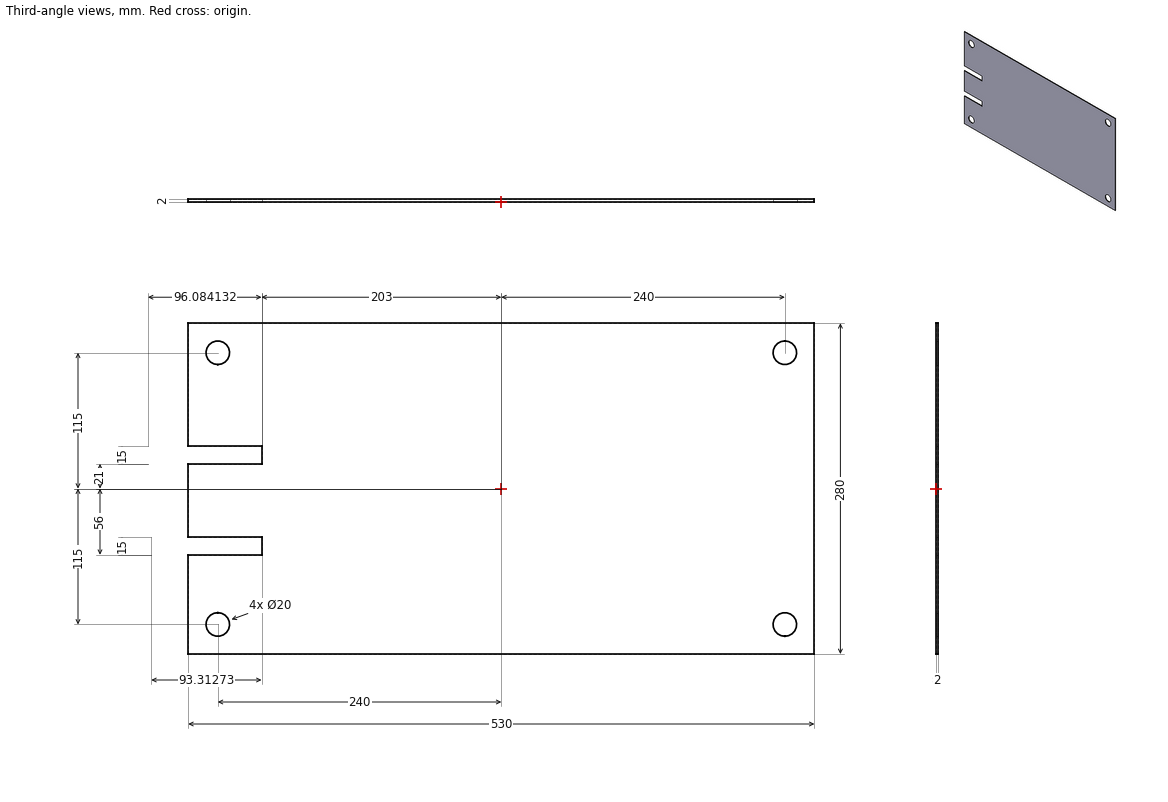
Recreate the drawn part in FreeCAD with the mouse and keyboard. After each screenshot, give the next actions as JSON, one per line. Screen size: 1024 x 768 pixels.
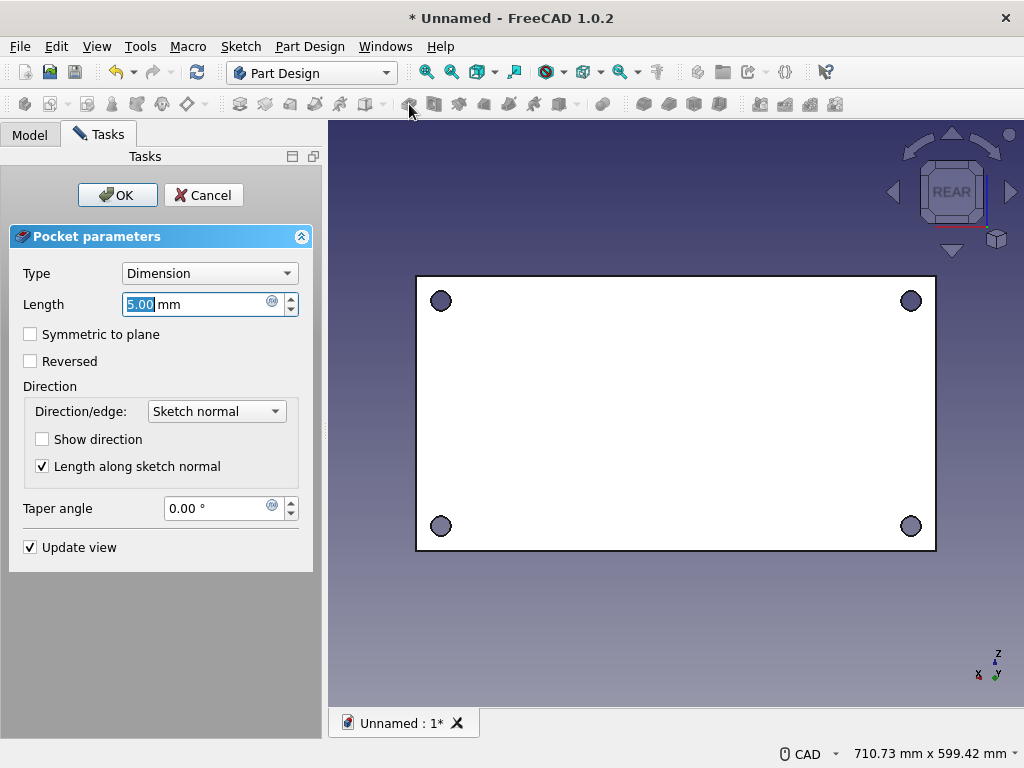
{"action": "type", "text": "2"}
{"action": "key", "text": "Tab"}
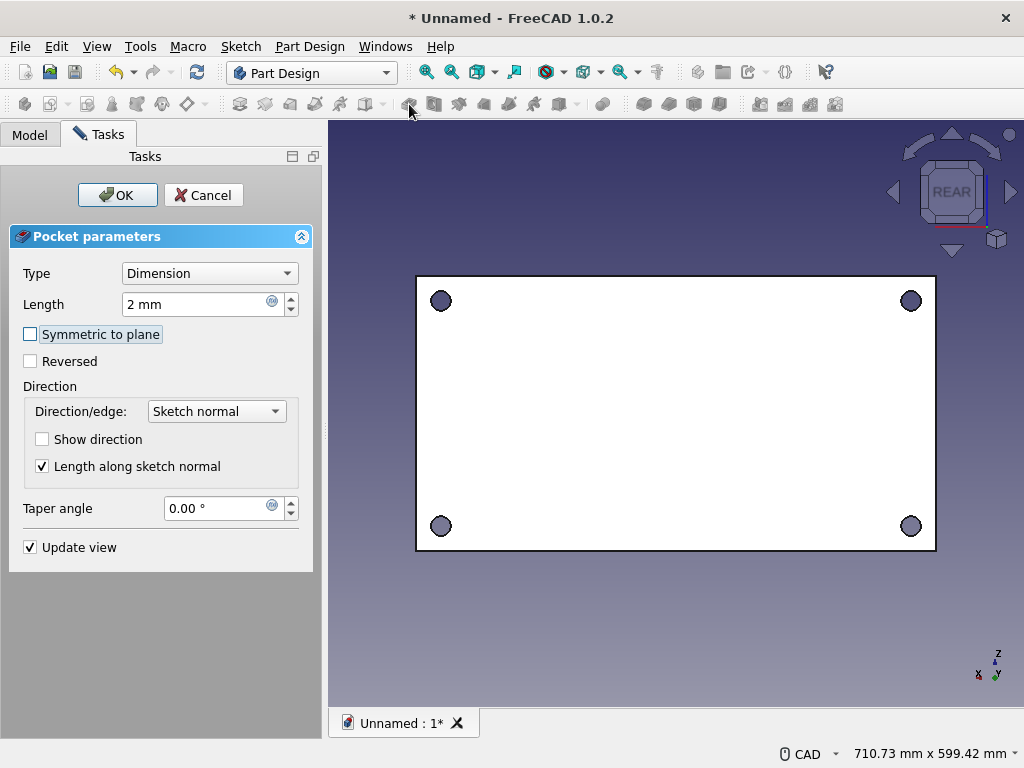
{"action": "left_click", "coordinate": [118, 195]}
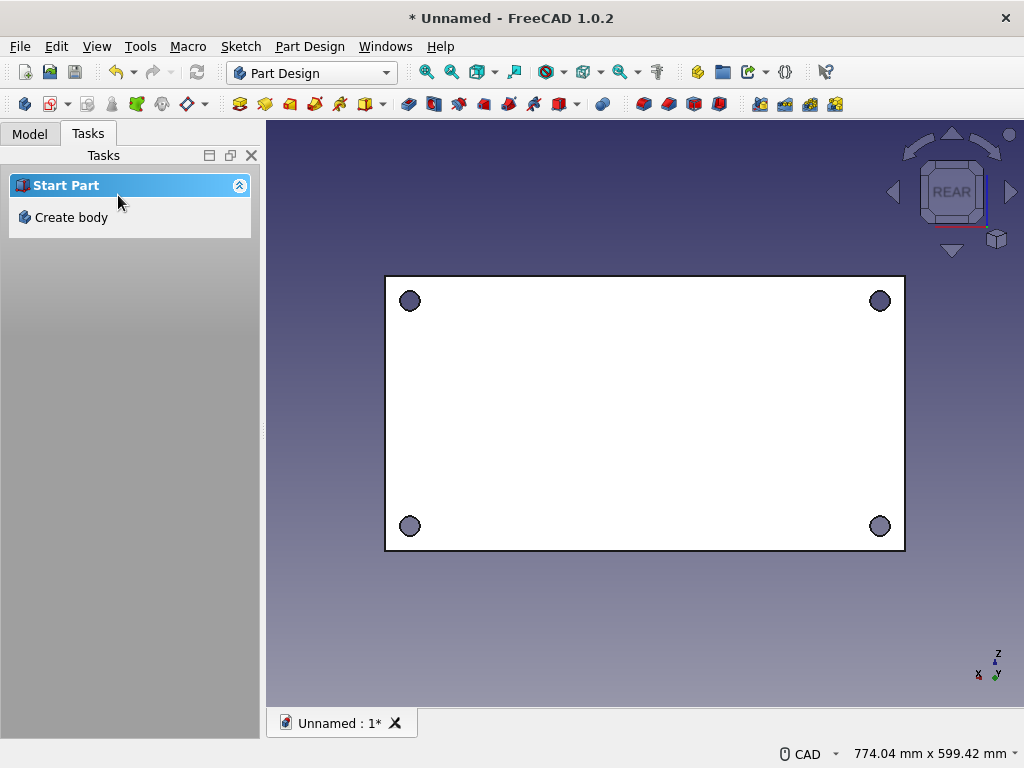
{"action": "left_click", "coordinate": [571, 412]}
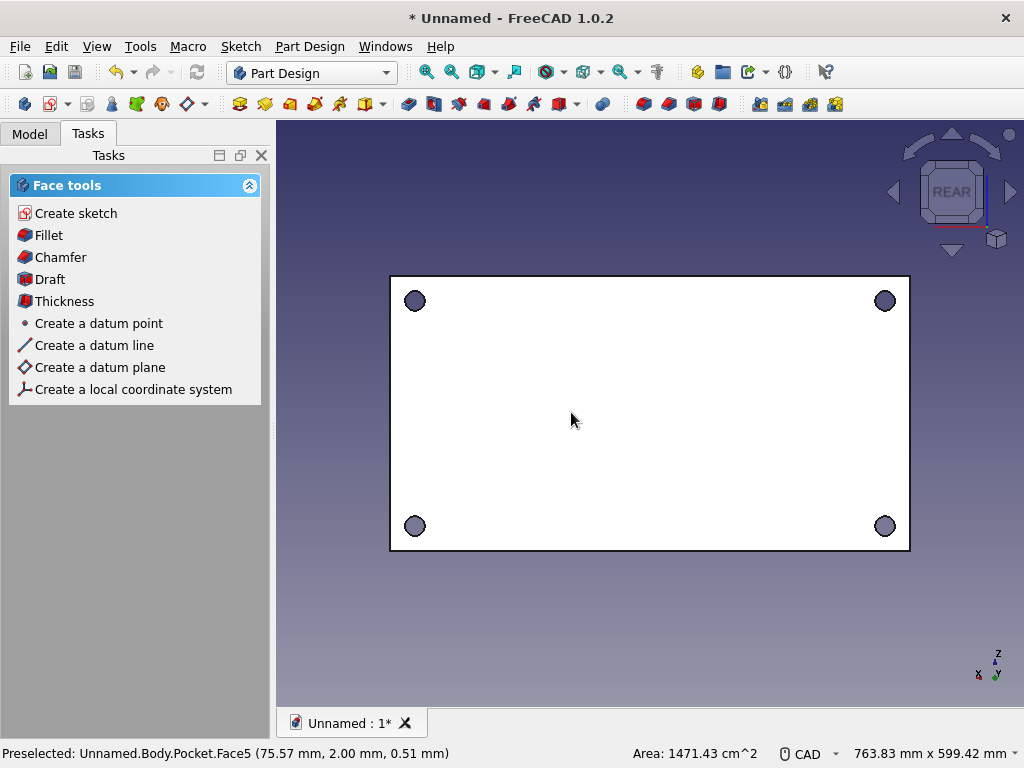
{"action": "left_click", "coordinate": [50, 104]}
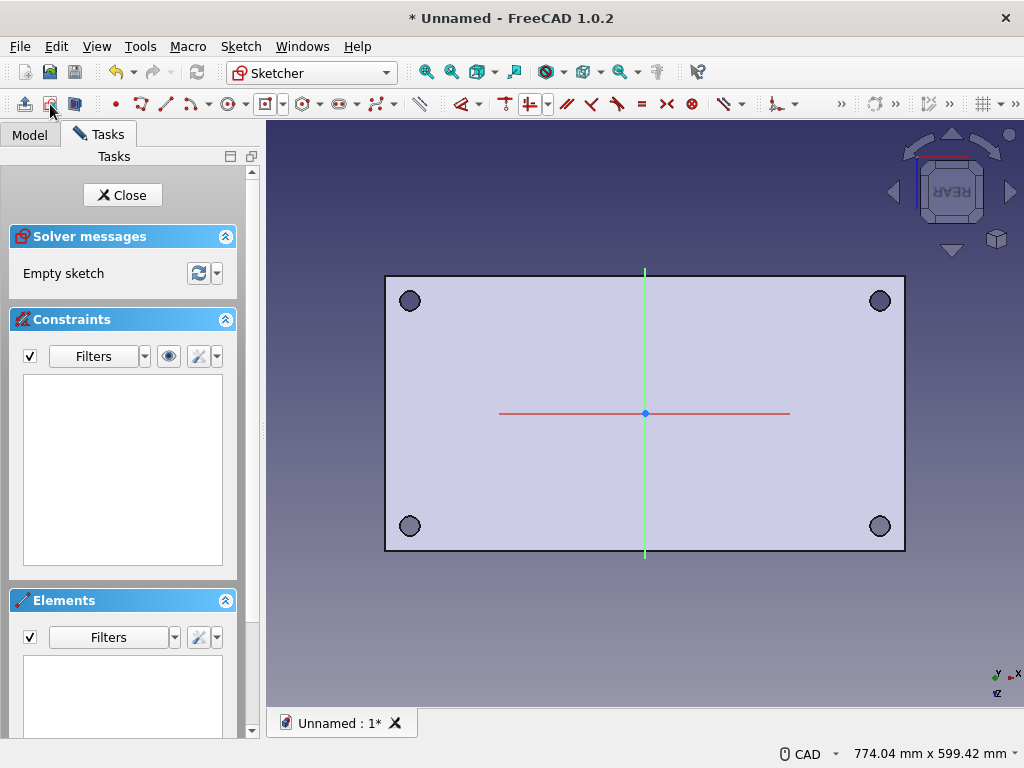
{"action": "scroll", "coordinate": [341, 401], "scroll_direction": "up", "scroll_amount": 7}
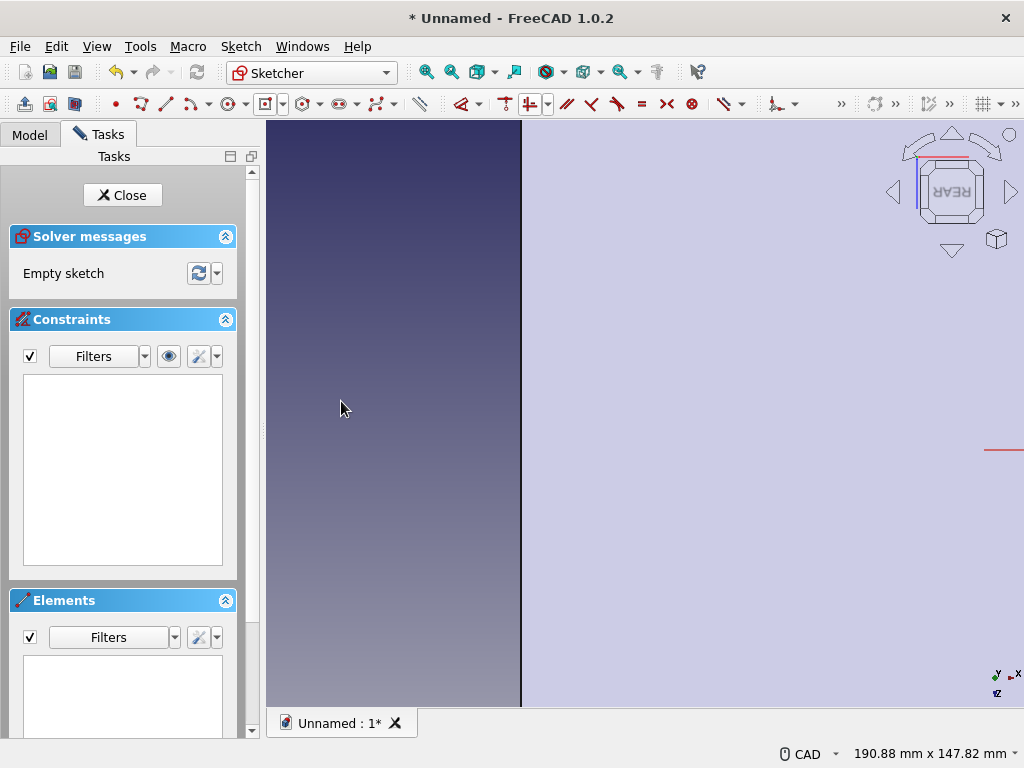
{"action": "key", "text": "g r"}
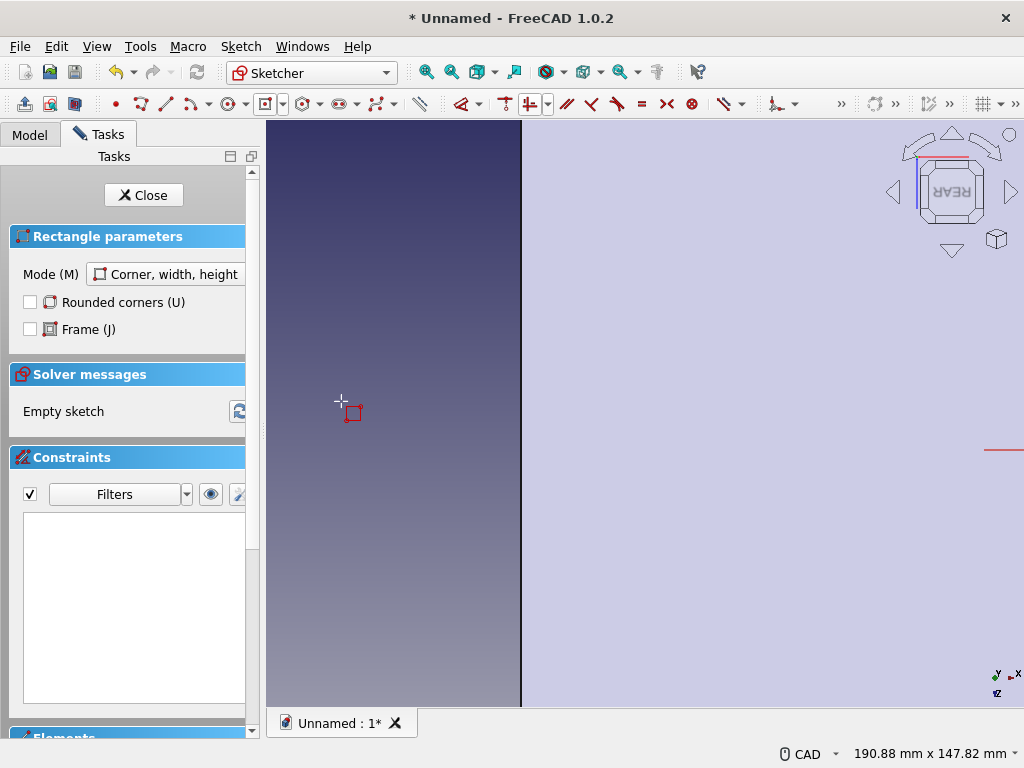
{"action": "left_click", "coordinate": [386, 534]}
{"action": "left_click", "coordinate": [767, 593]}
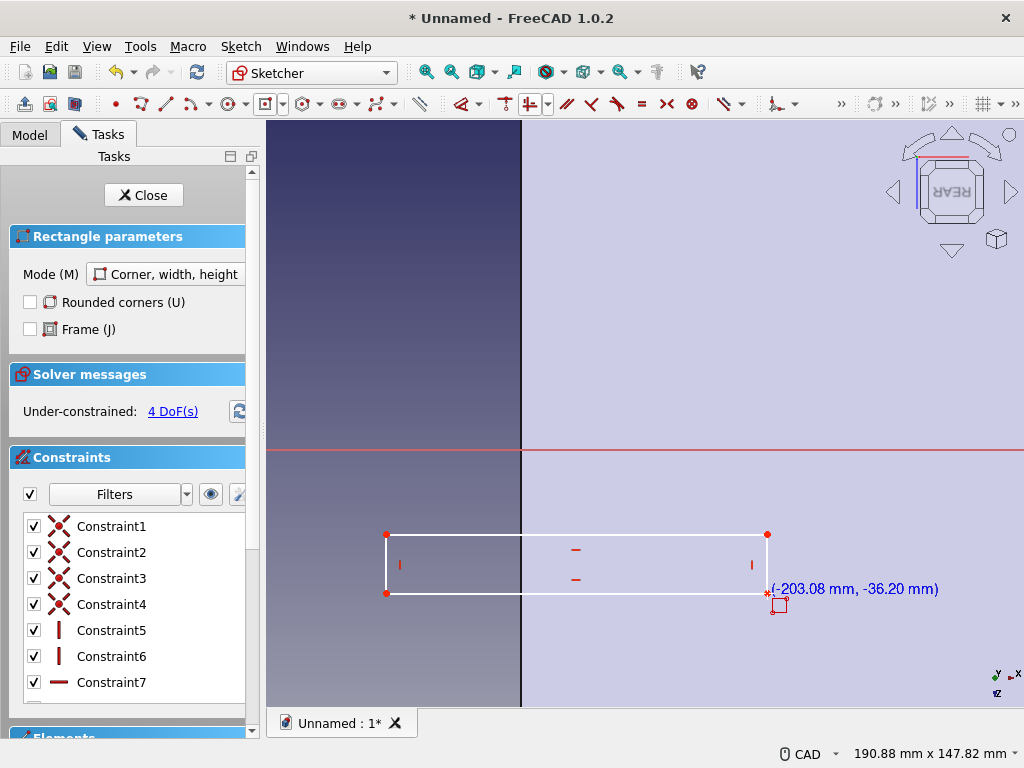
{"action": "left_click", "coordinate": [397, 228]}
{"action": "left_click", "coordinate": [767, 287]}
{"action": "key", "text": "Escape"}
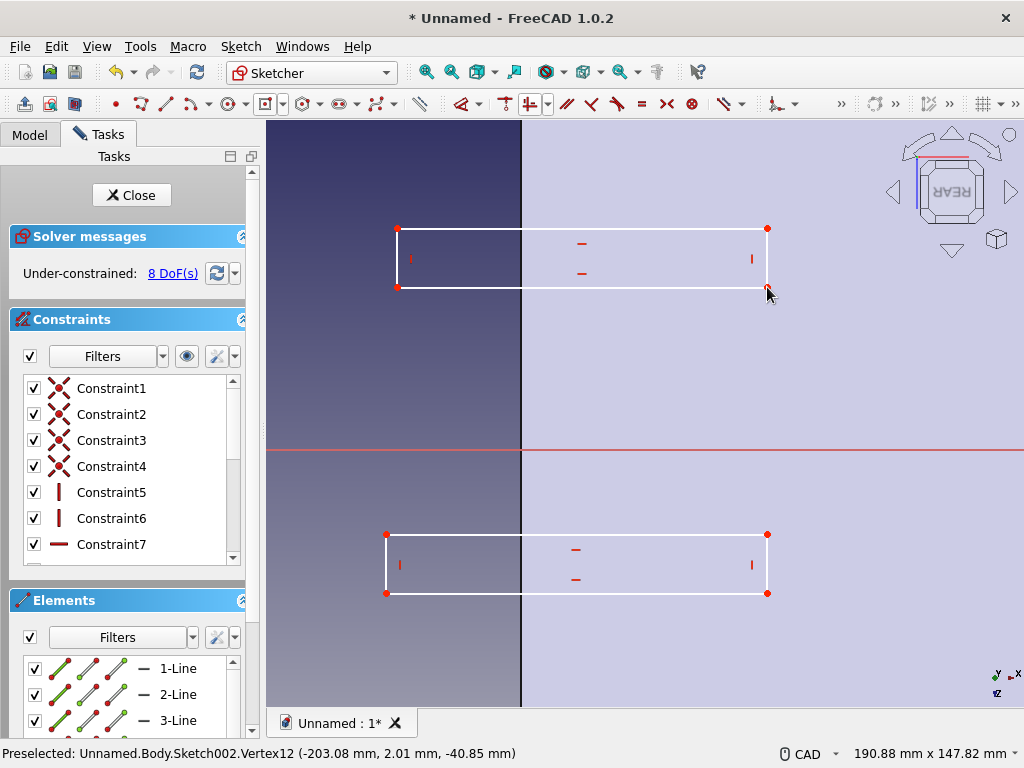
{"action": "left_click", "coordinate": [460, 104]}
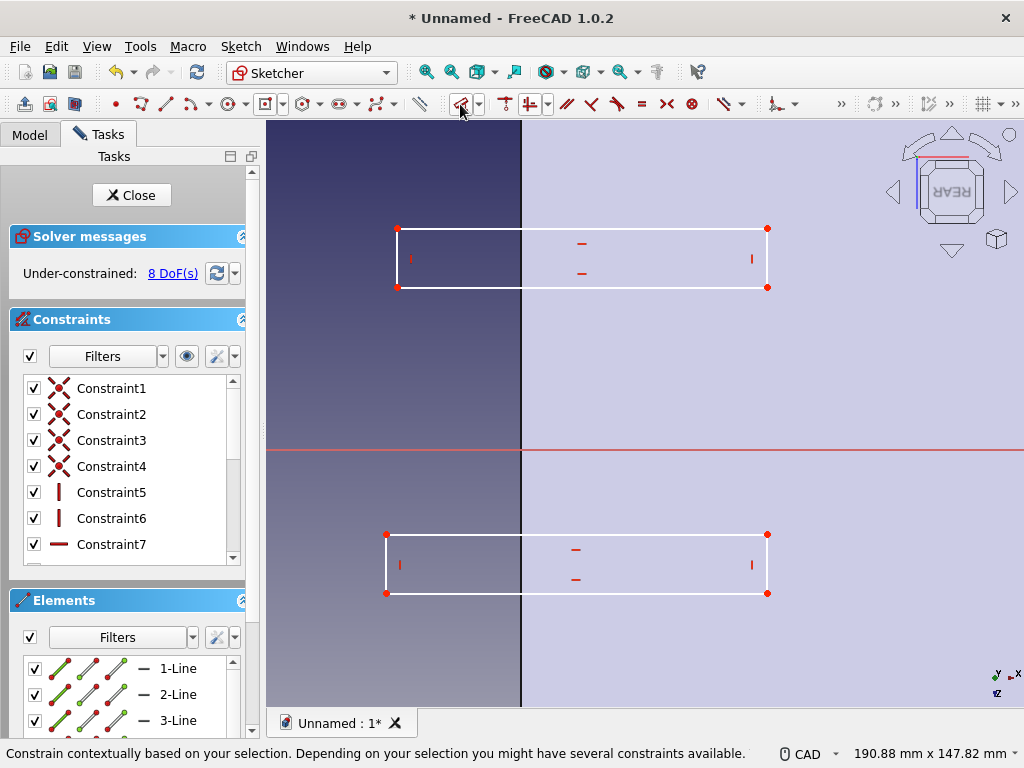
{"action": "left_click", "coordinate": [386, 553]}
{"action": "left_click", "coordinate": [352, 565]}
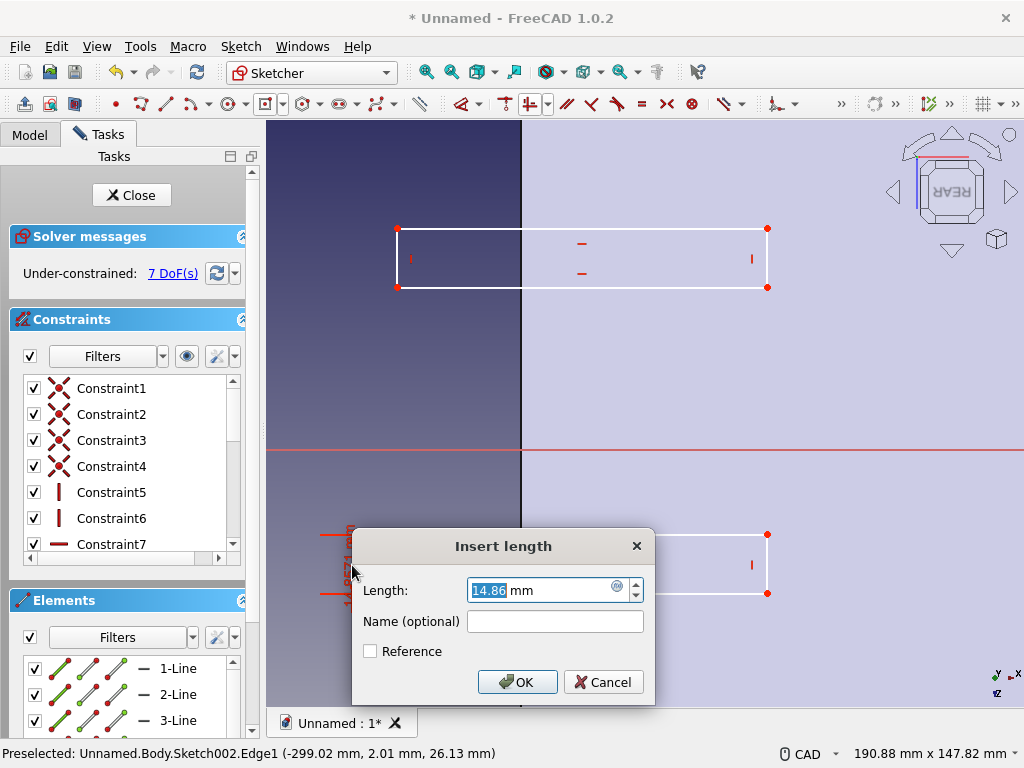
{"action": "type", "text": "15"}
{"action": "key", "text": "Return"}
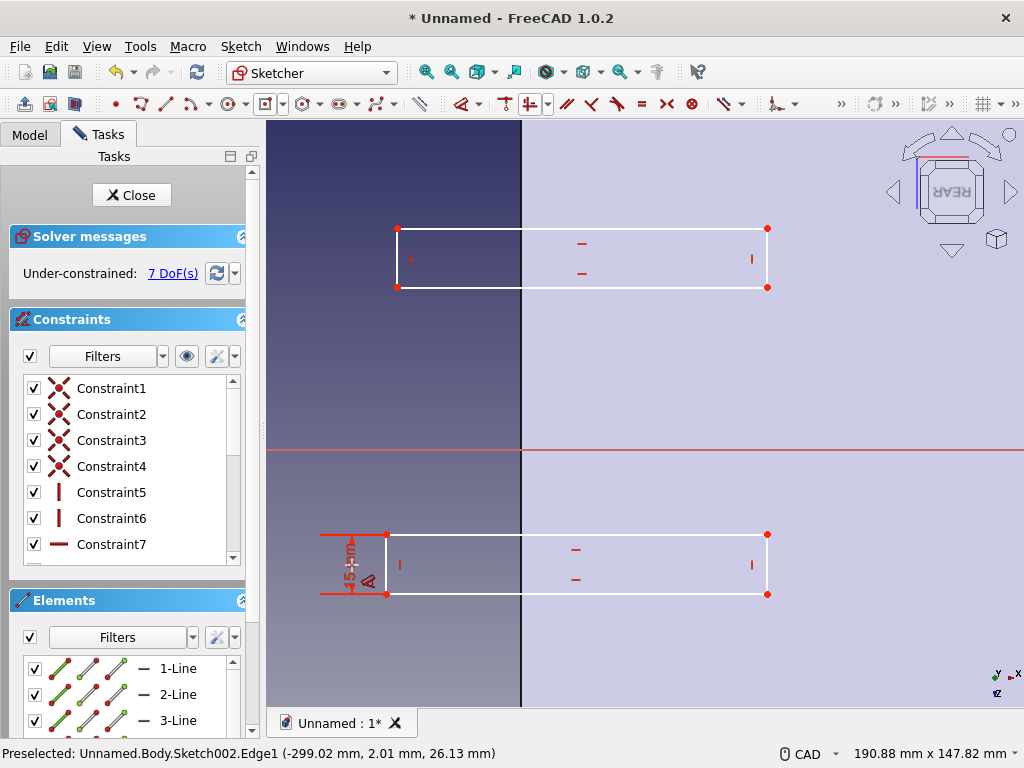
{"action": "left_click", "coordinate": [397, 247]}
{"action": "left_click", "coordinate": [363, 258]}